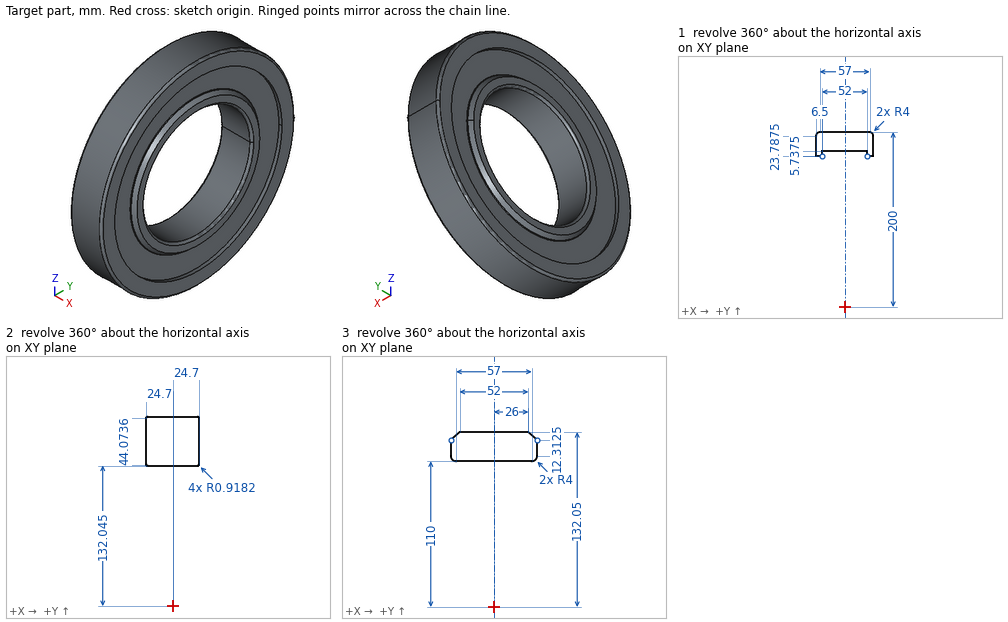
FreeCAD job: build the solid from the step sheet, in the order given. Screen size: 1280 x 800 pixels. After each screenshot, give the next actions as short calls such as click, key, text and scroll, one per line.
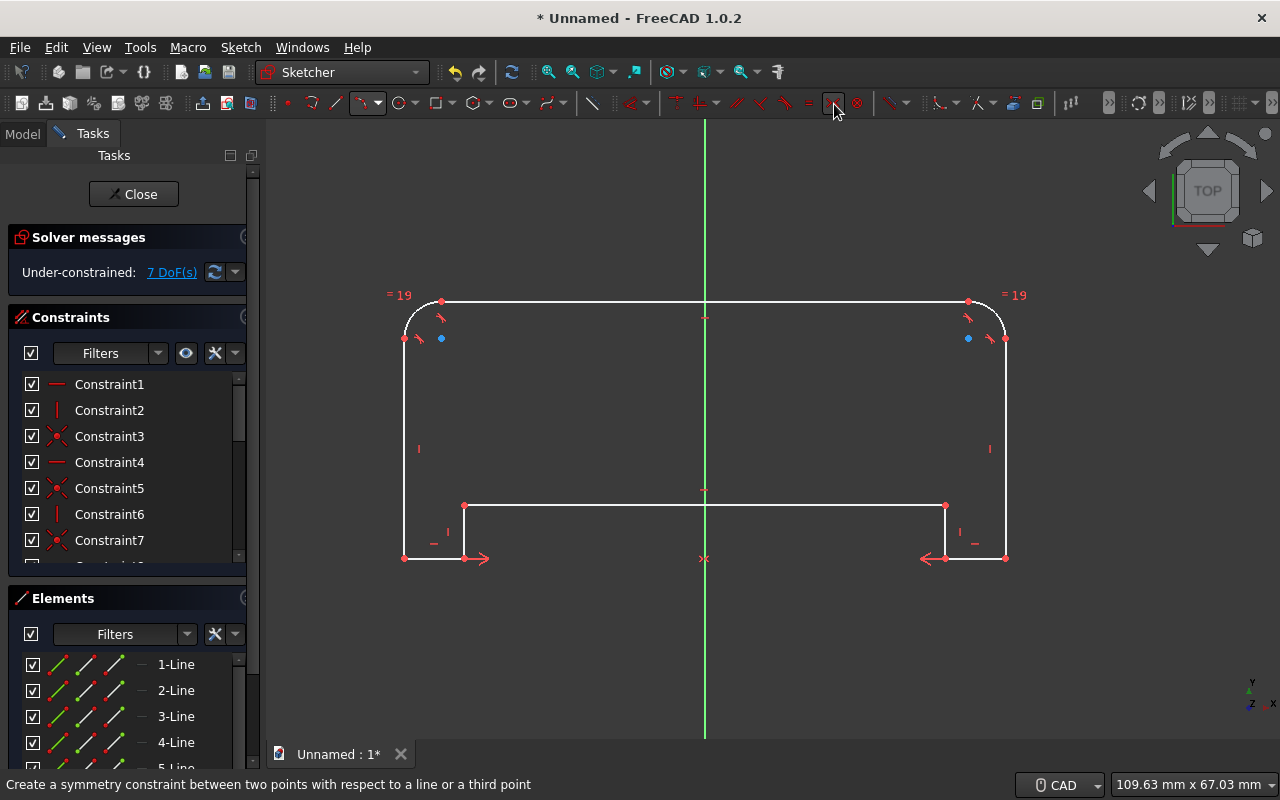
click(630, 104)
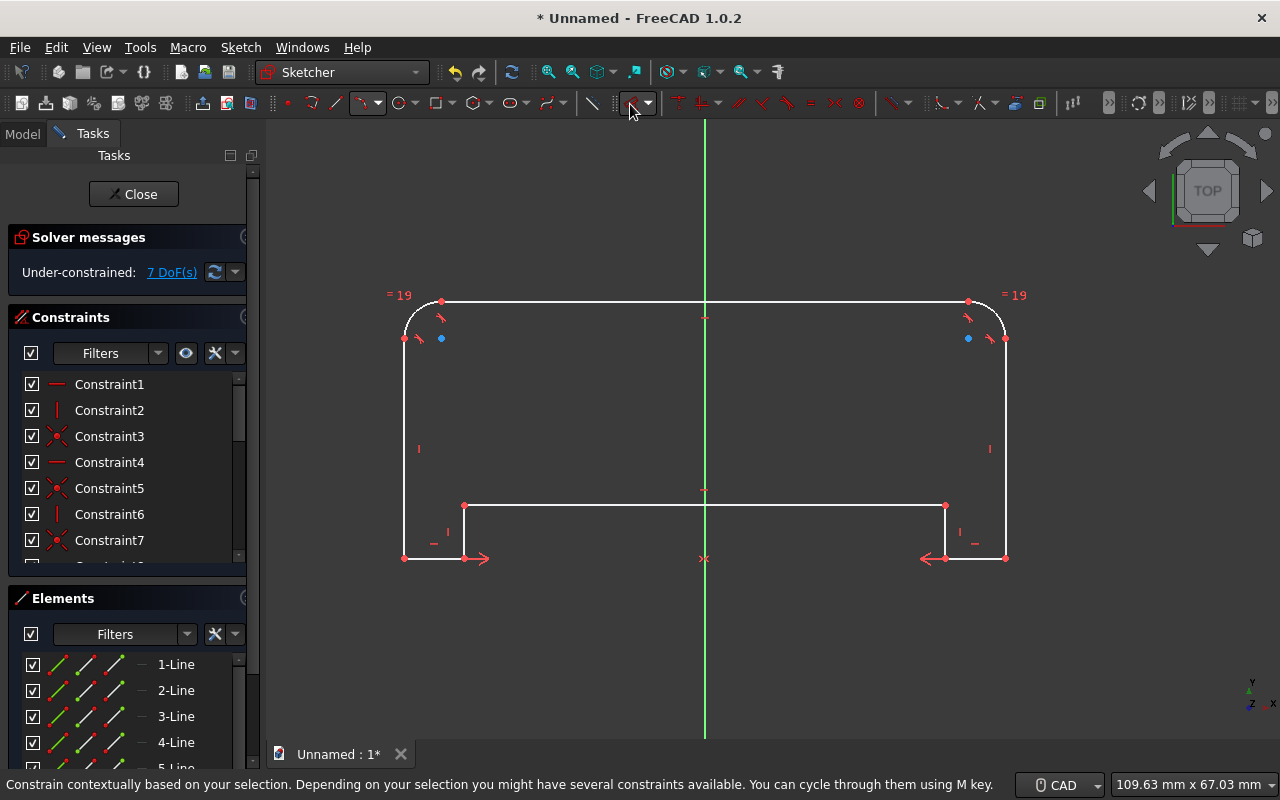
click(425, 306)
click(411, 277)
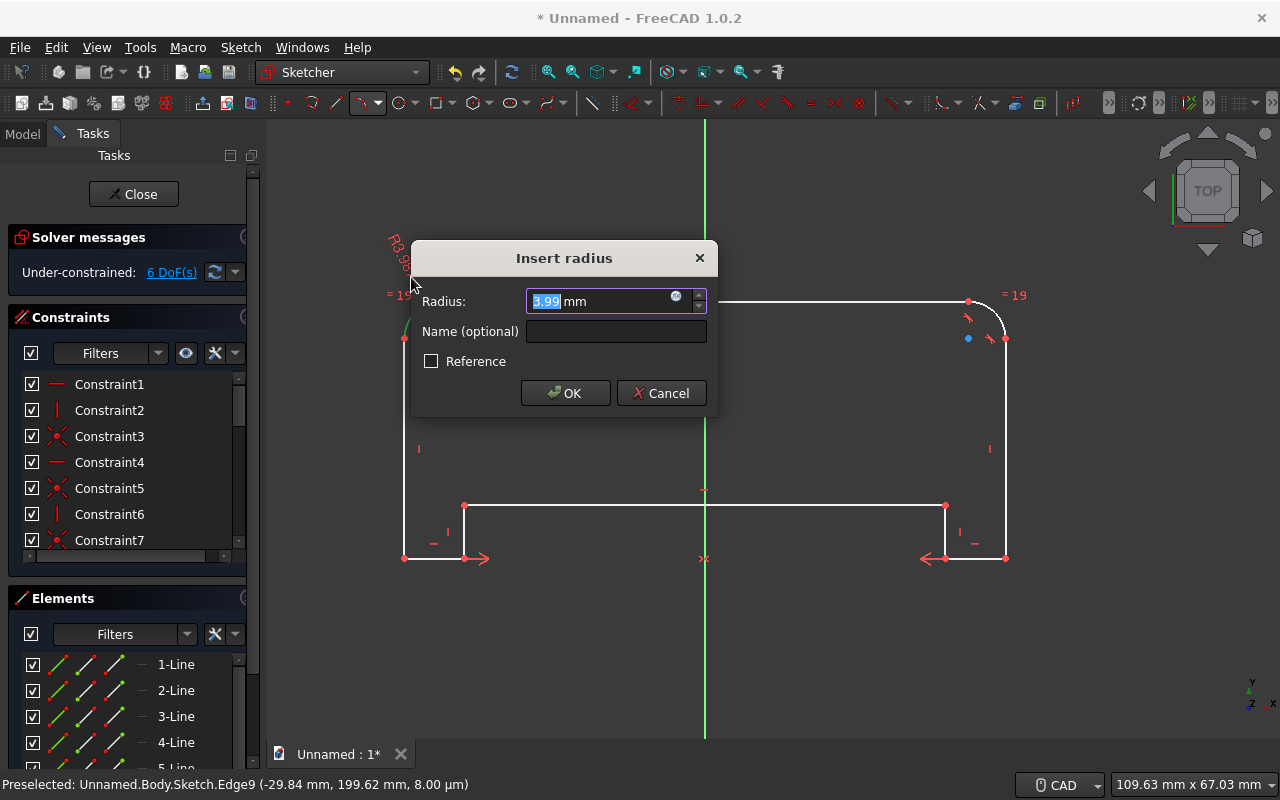
text(4)
key(Return)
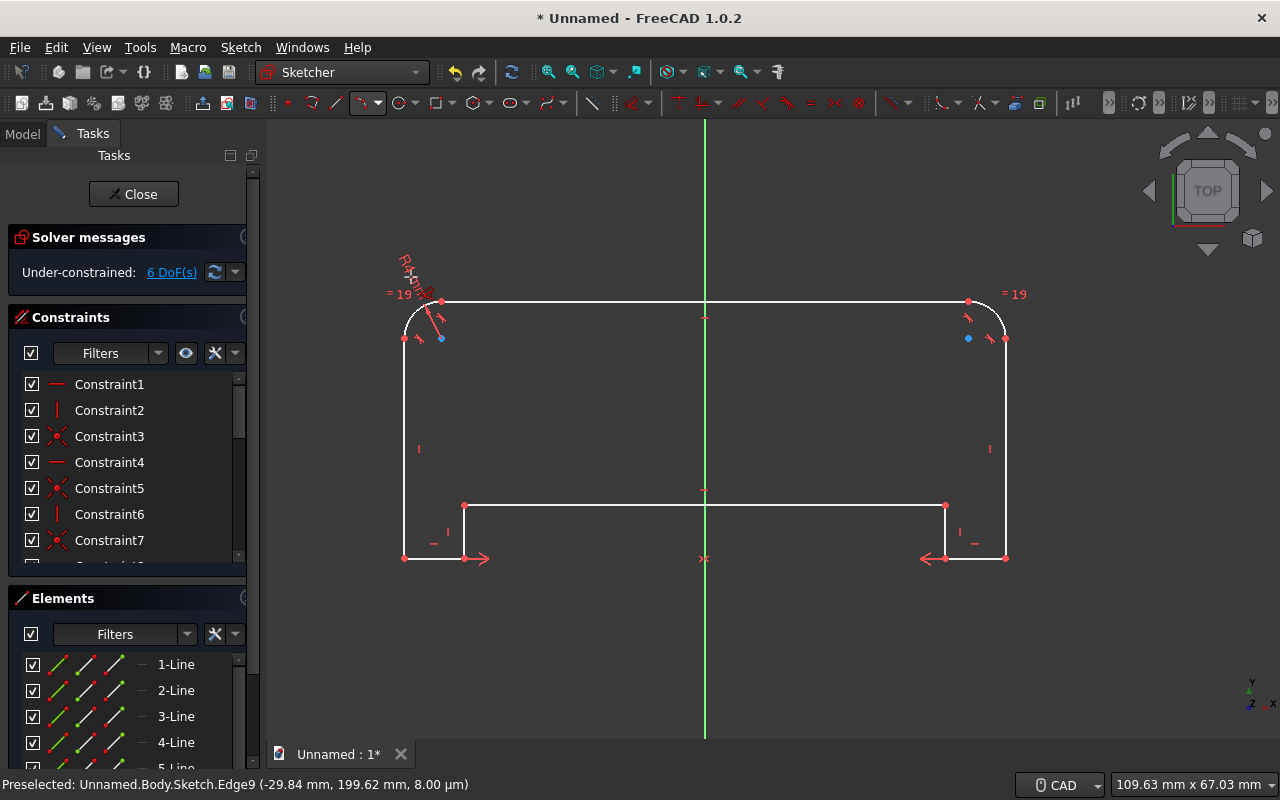
click(810, 302)
click(584, 268)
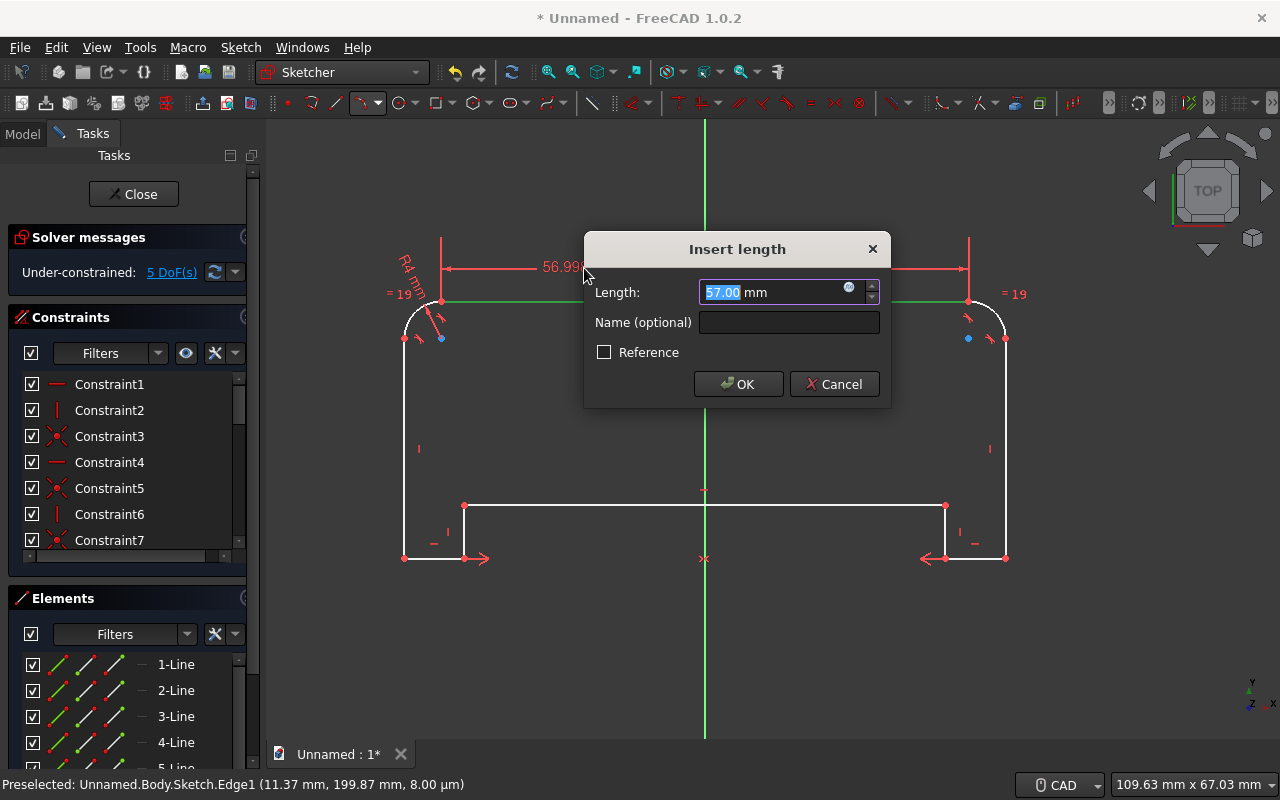
text(57)
key(Return)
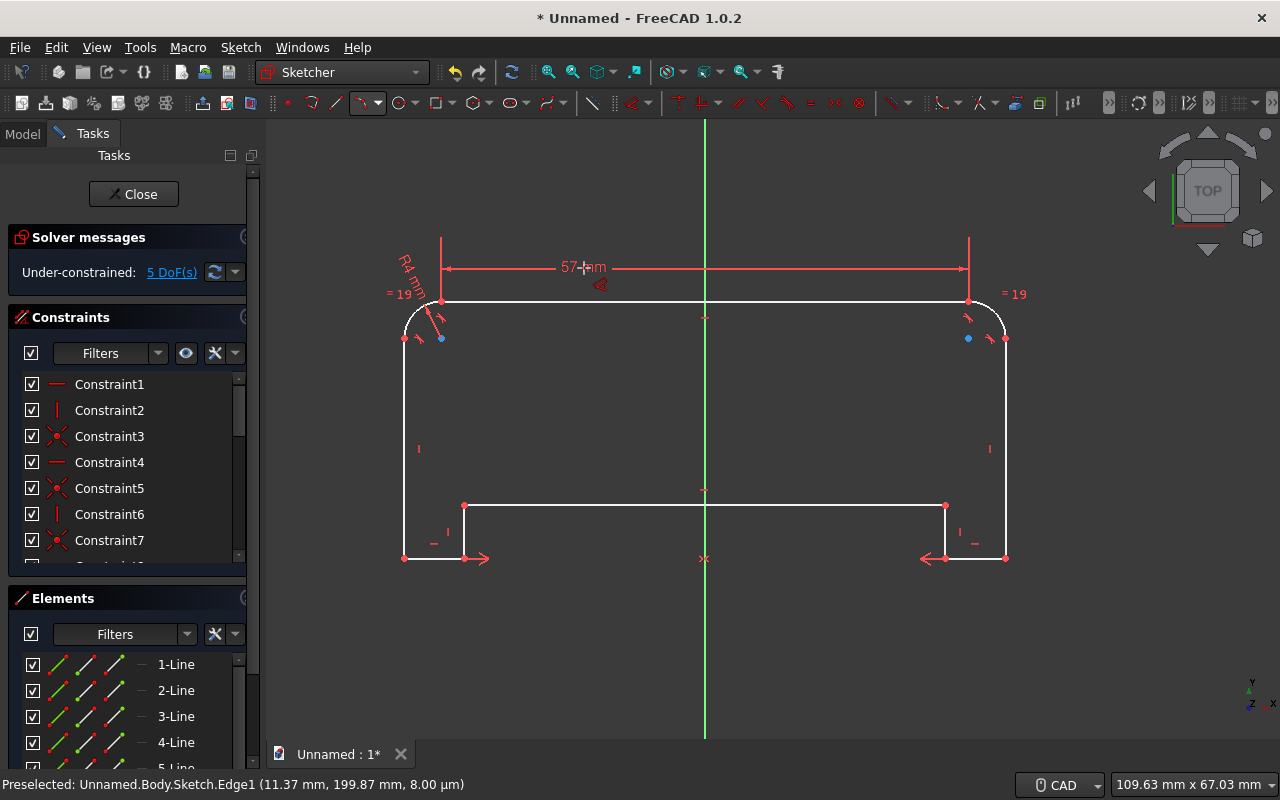
click(609, 505)
click(594, 539)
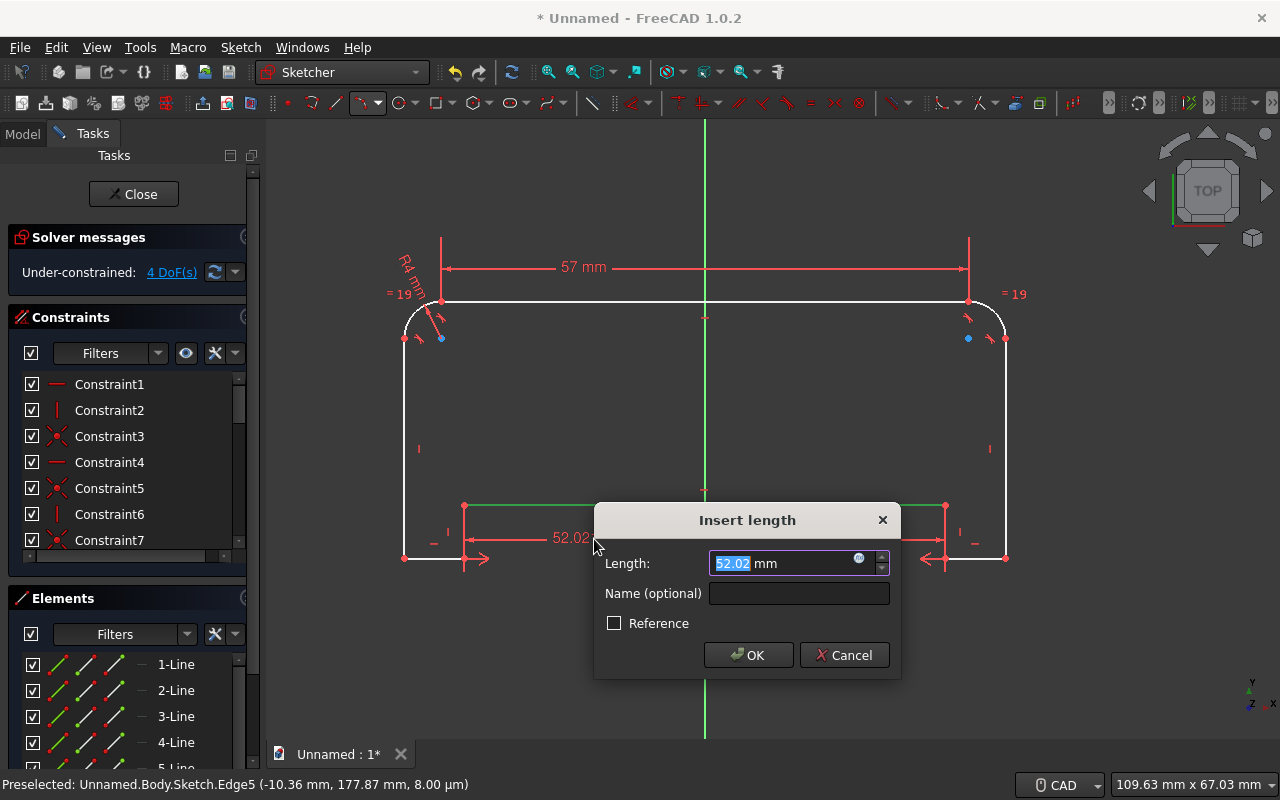
text(52)
key(Return)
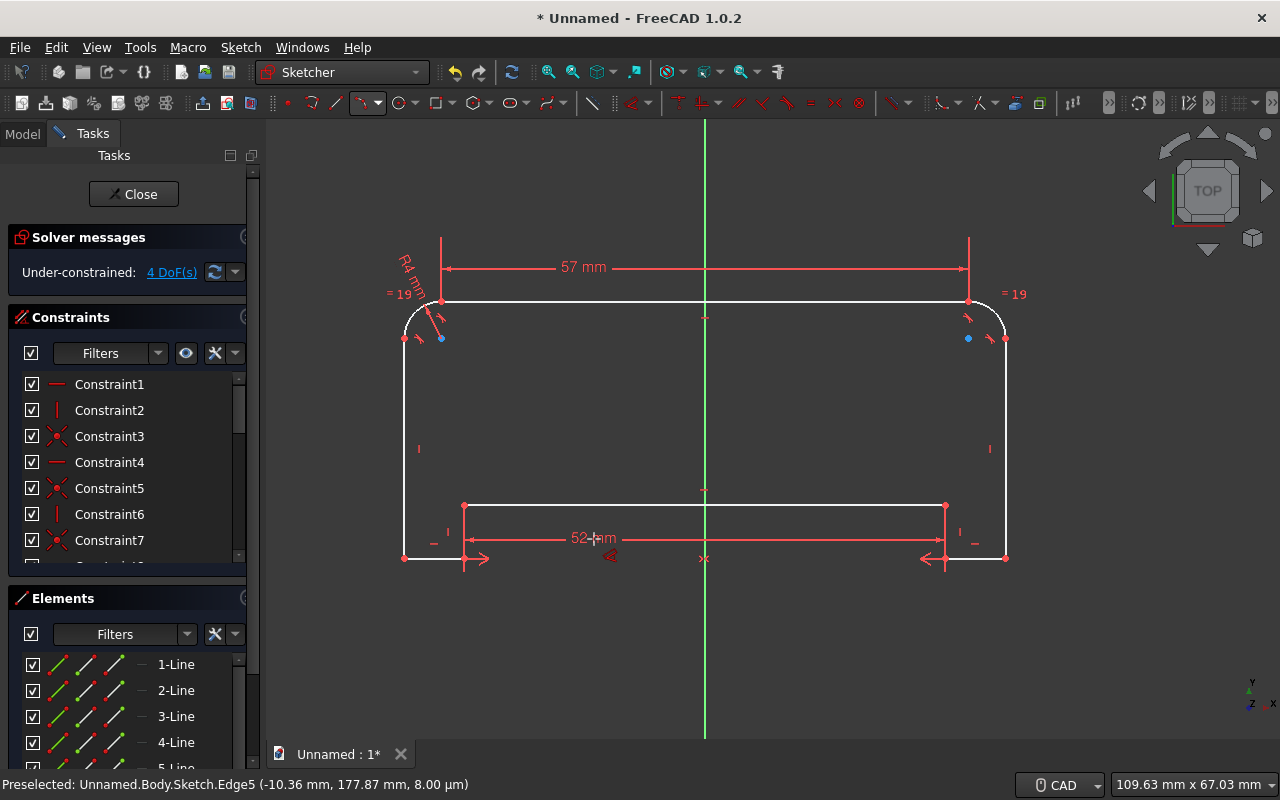
click(422, 559)
click(434, 593)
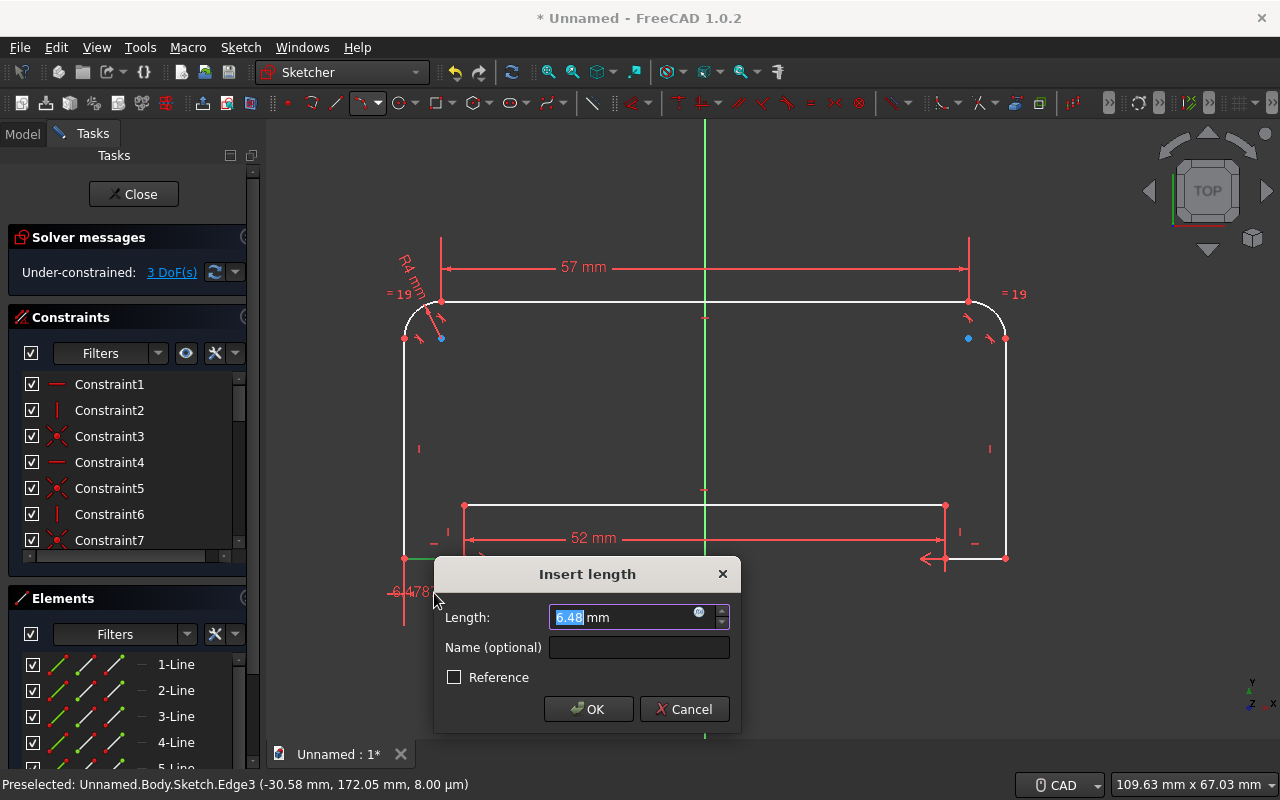
text(6.5)
key(Return)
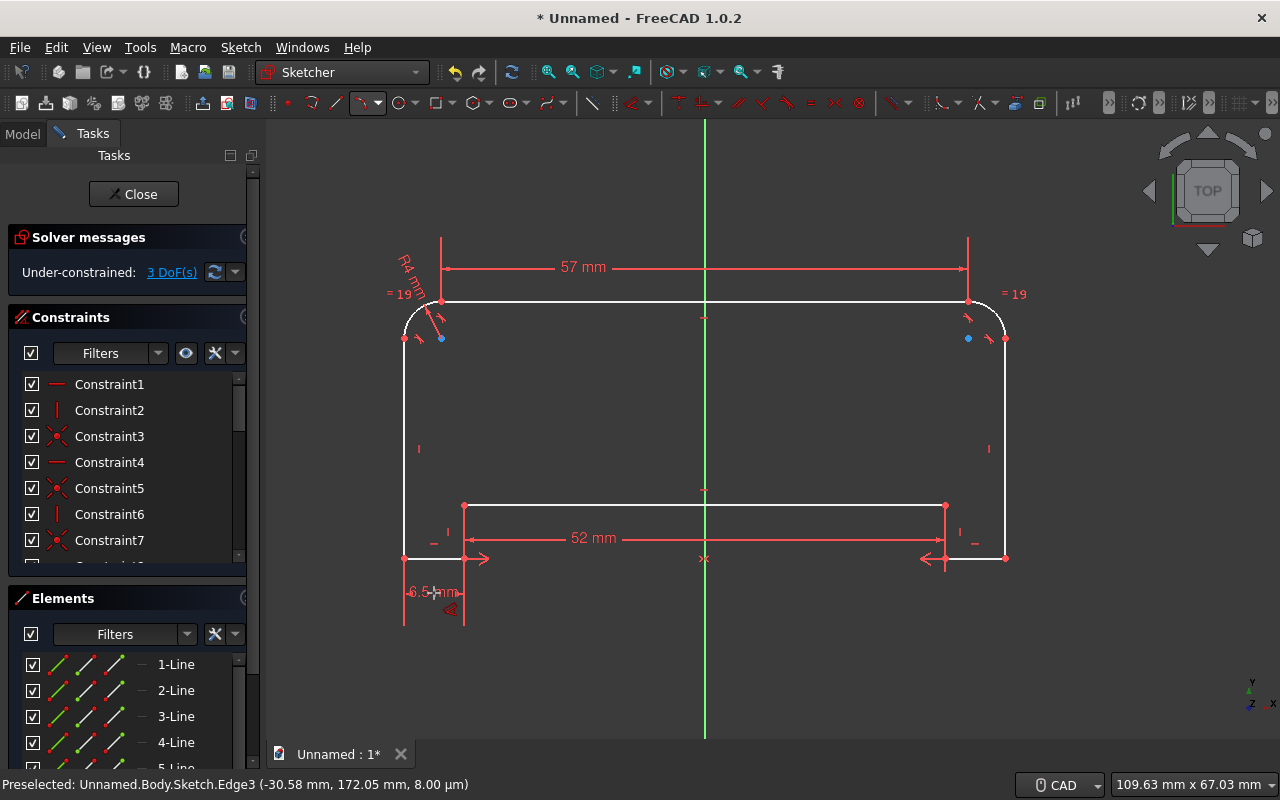
click(968, 302)
click(1002, 600)